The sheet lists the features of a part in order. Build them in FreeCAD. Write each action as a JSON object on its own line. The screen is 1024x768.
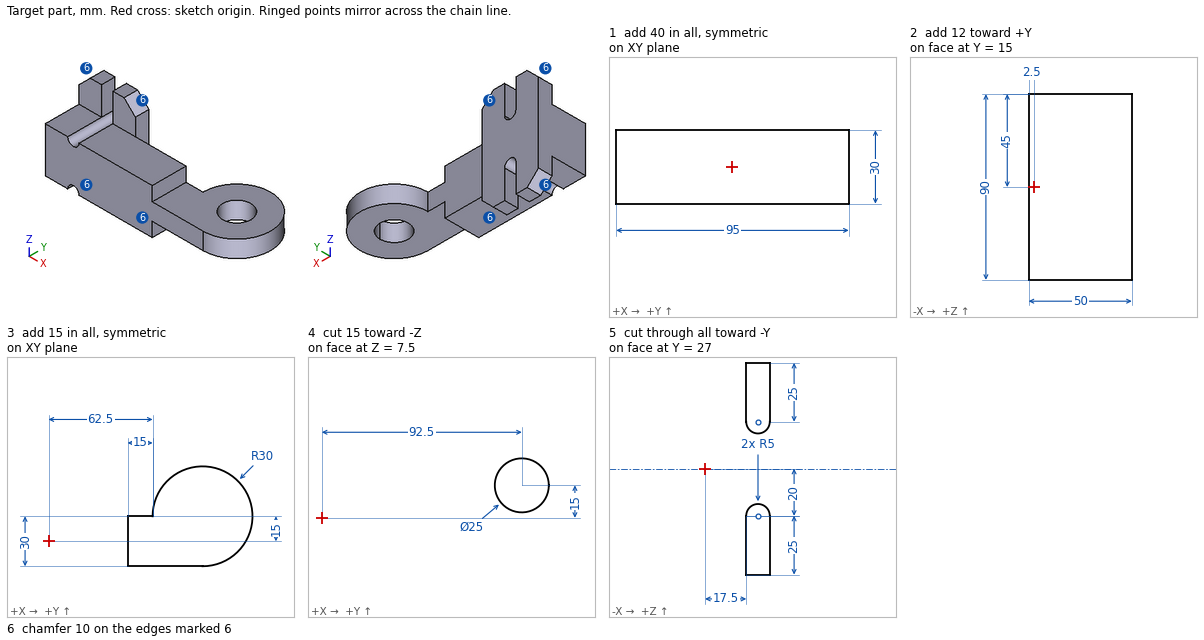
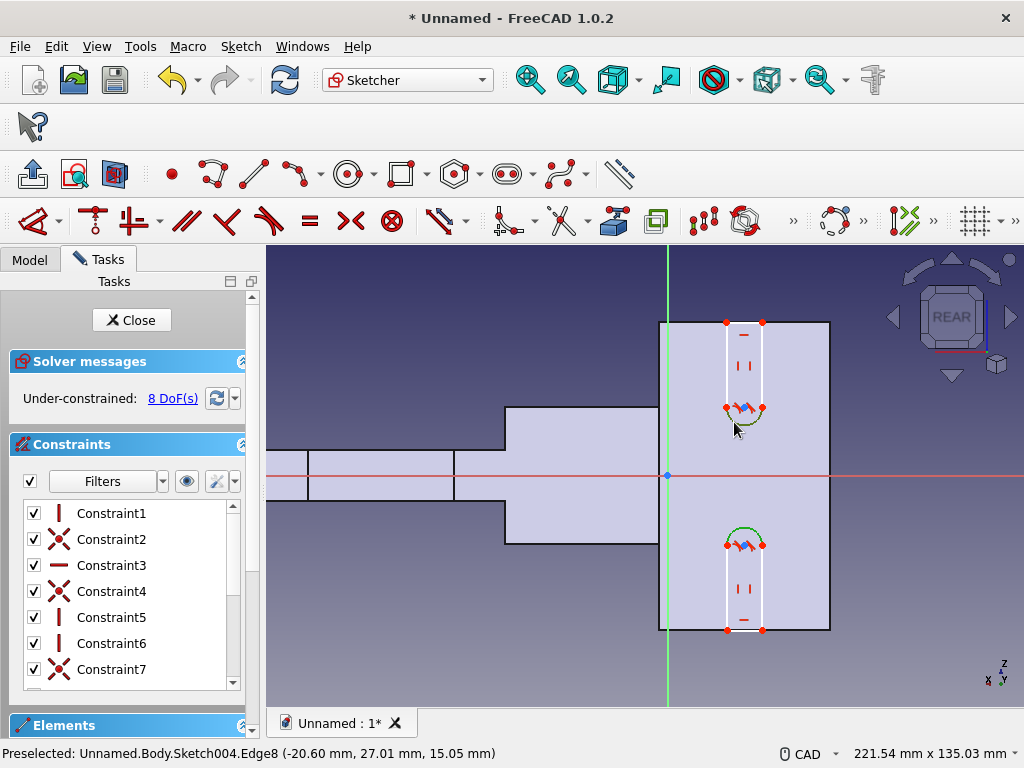
{"action": "left_click", "coordinate": [310, 222]}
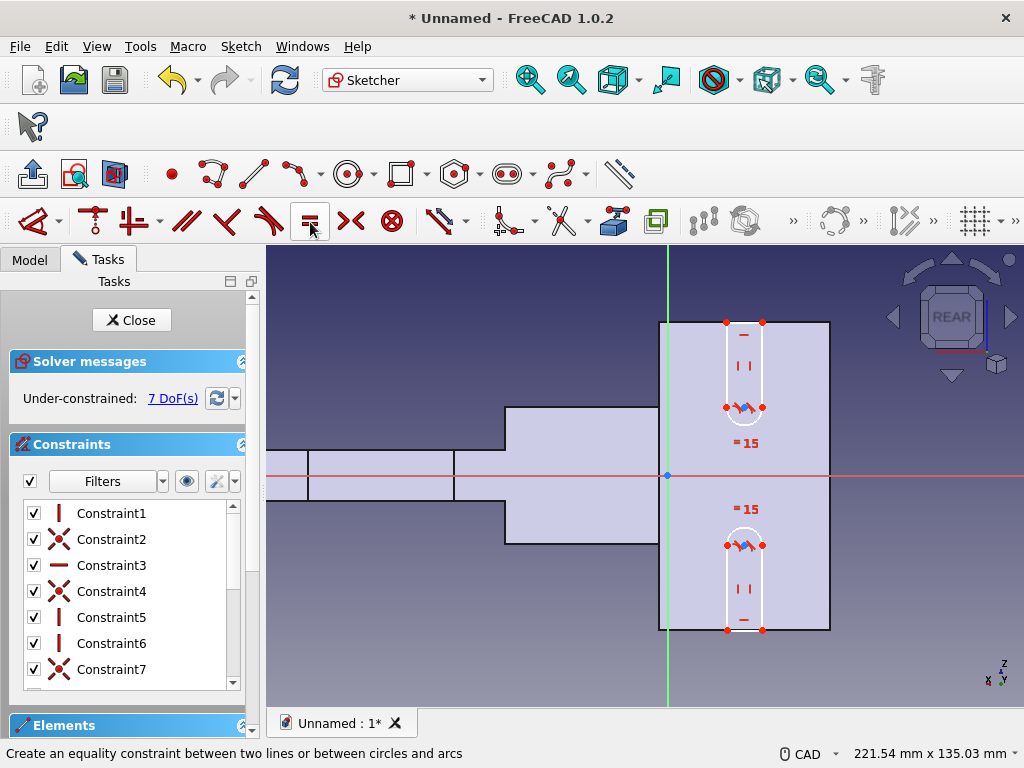
{"action": "left_click", "coordinate": [745, 545]}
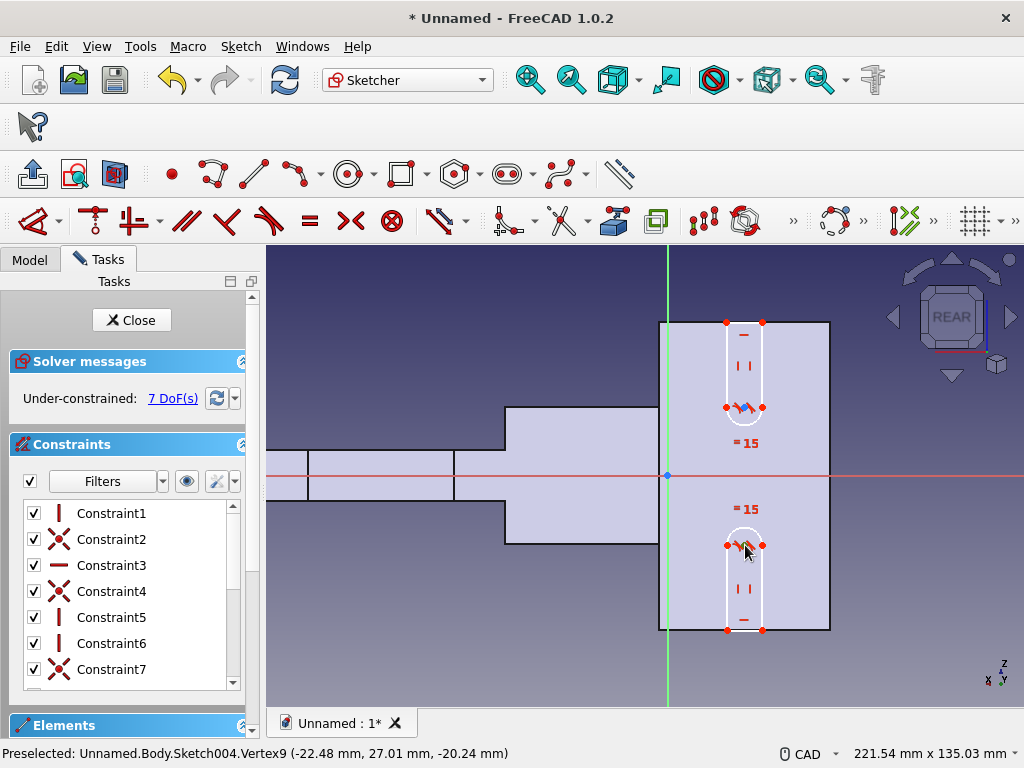
{"action": "left_click", "coordinate": [744, 408]}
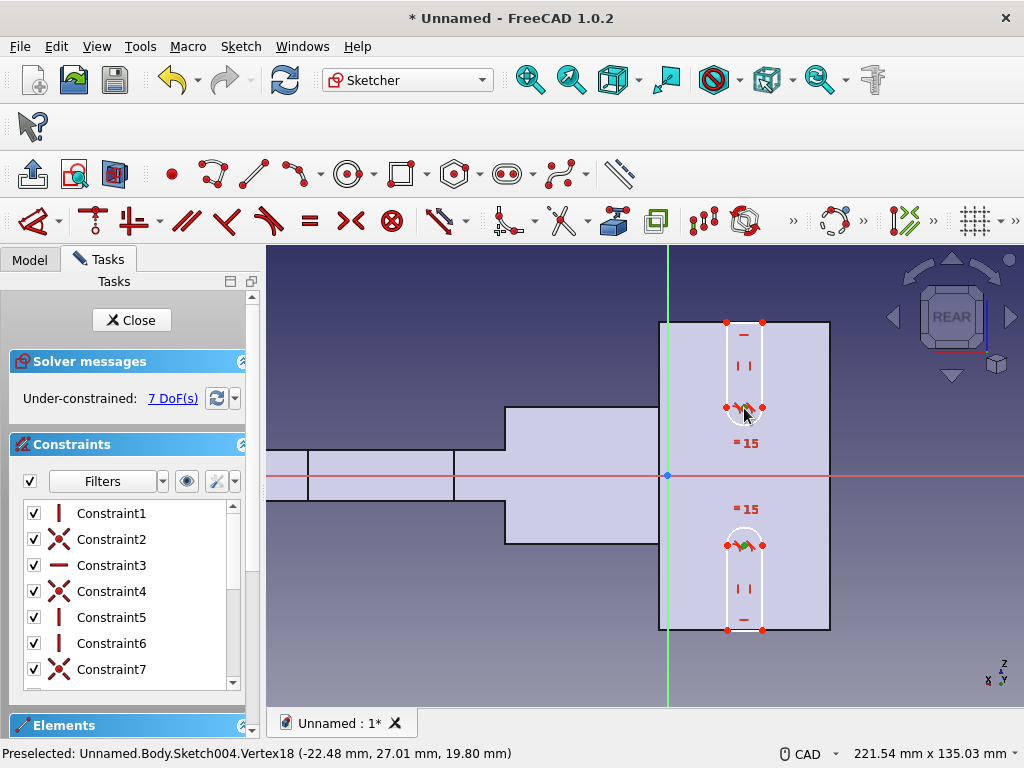
{"action": "left_click", "coordinate": [334, 476]}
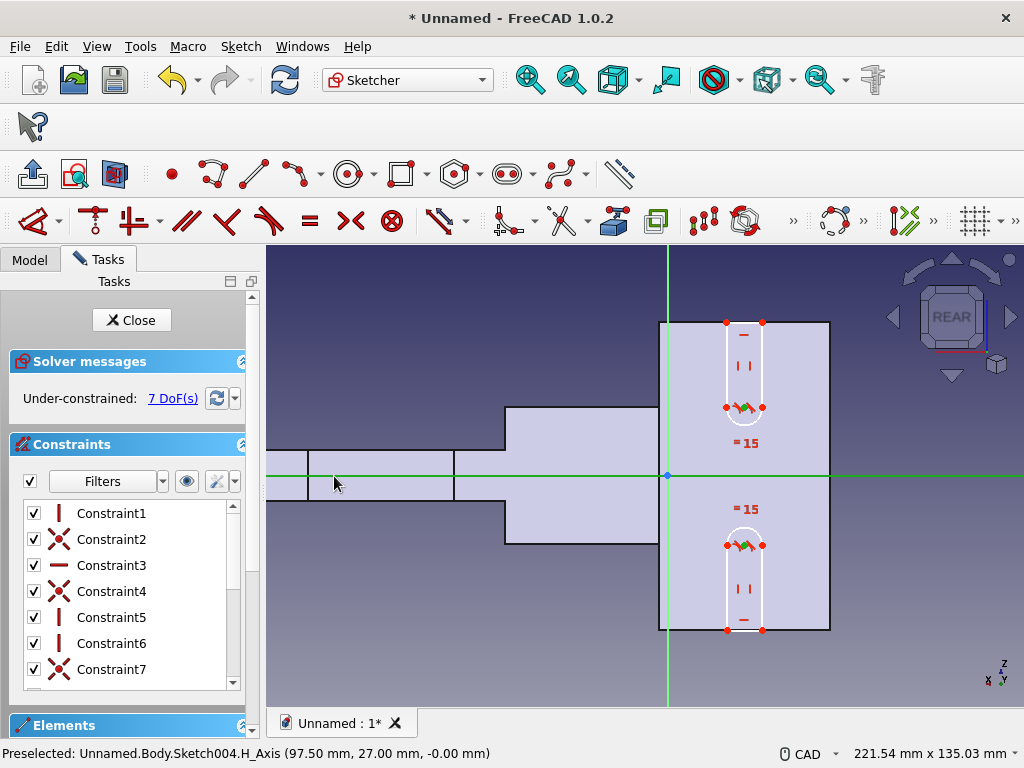
{"action": "key", "text": "s"}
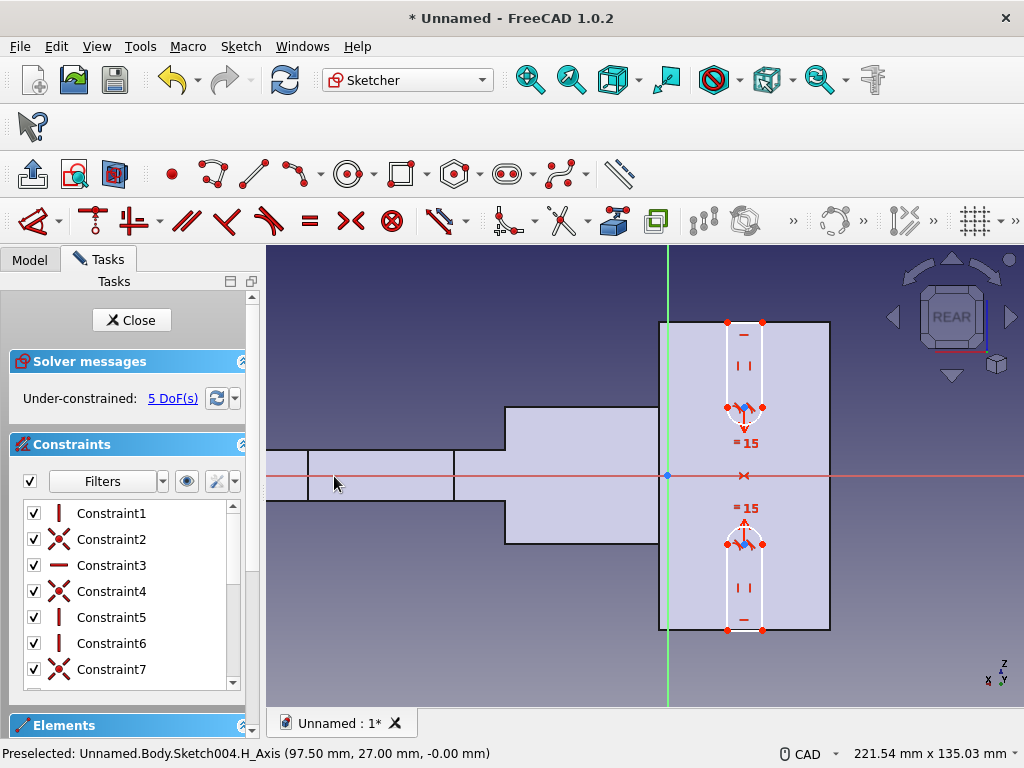
{"action": "left_click", "coordinate": [32, 222]}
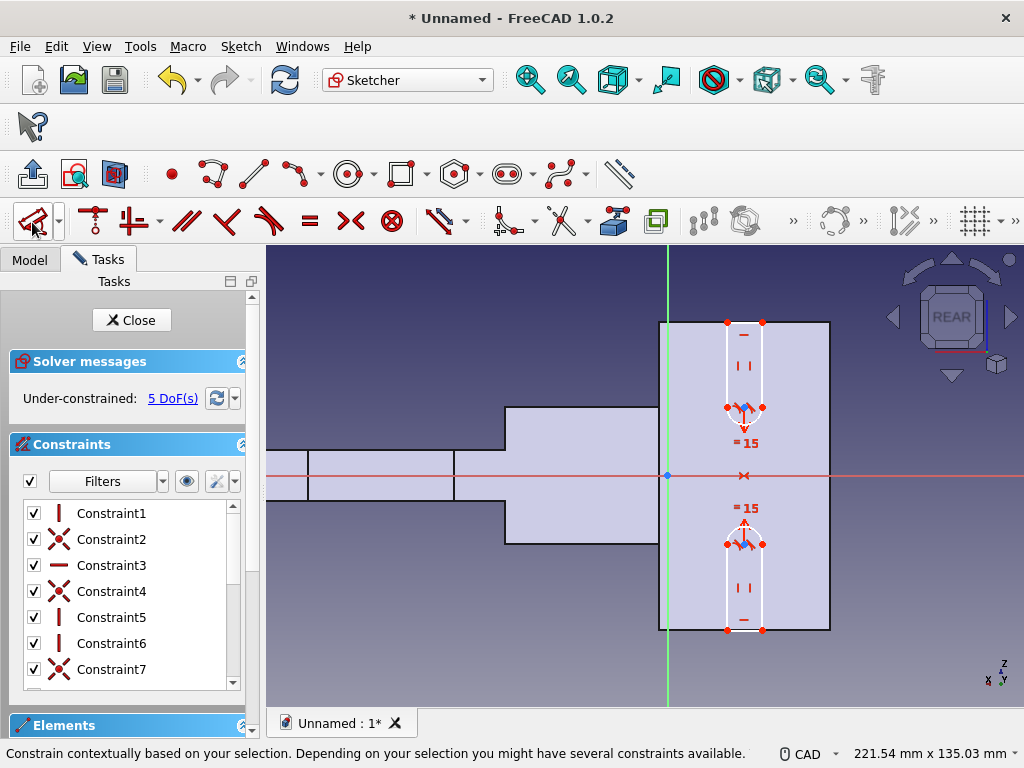
{"action": "scroll", "coordinate": [755, 530], "scroll_direction": "up", "scroll_amount": 5}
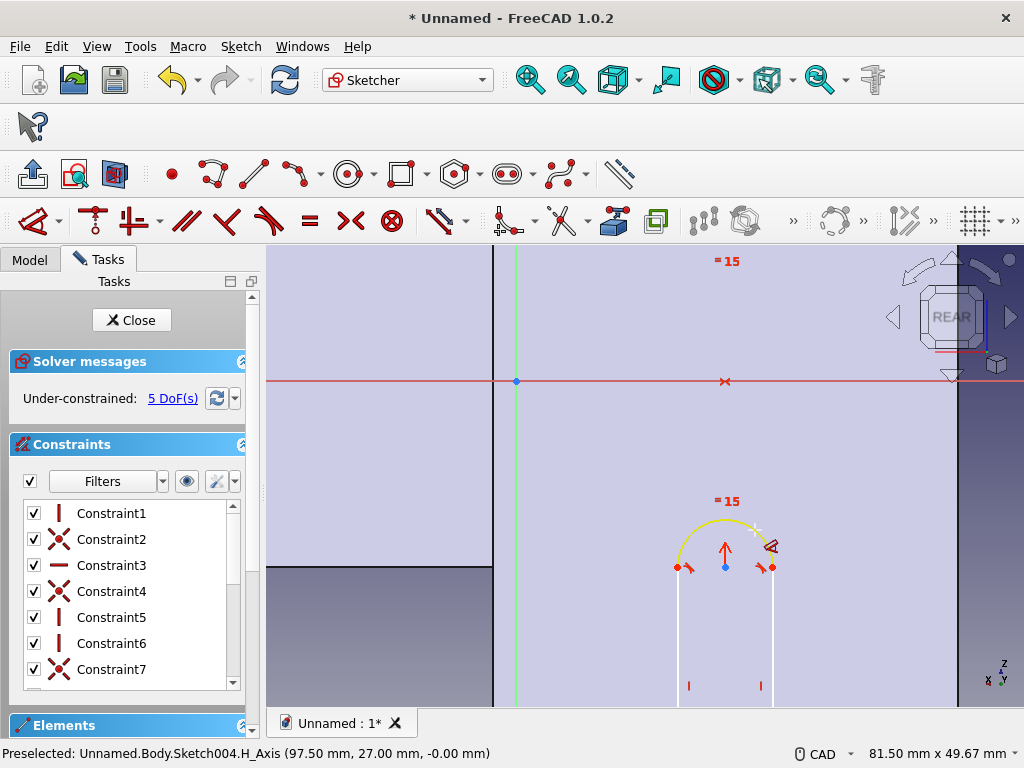
{"action": "left_click", "coordinate": [753, 529]}
{"action": "left_click", "coordinate": [772, 503]}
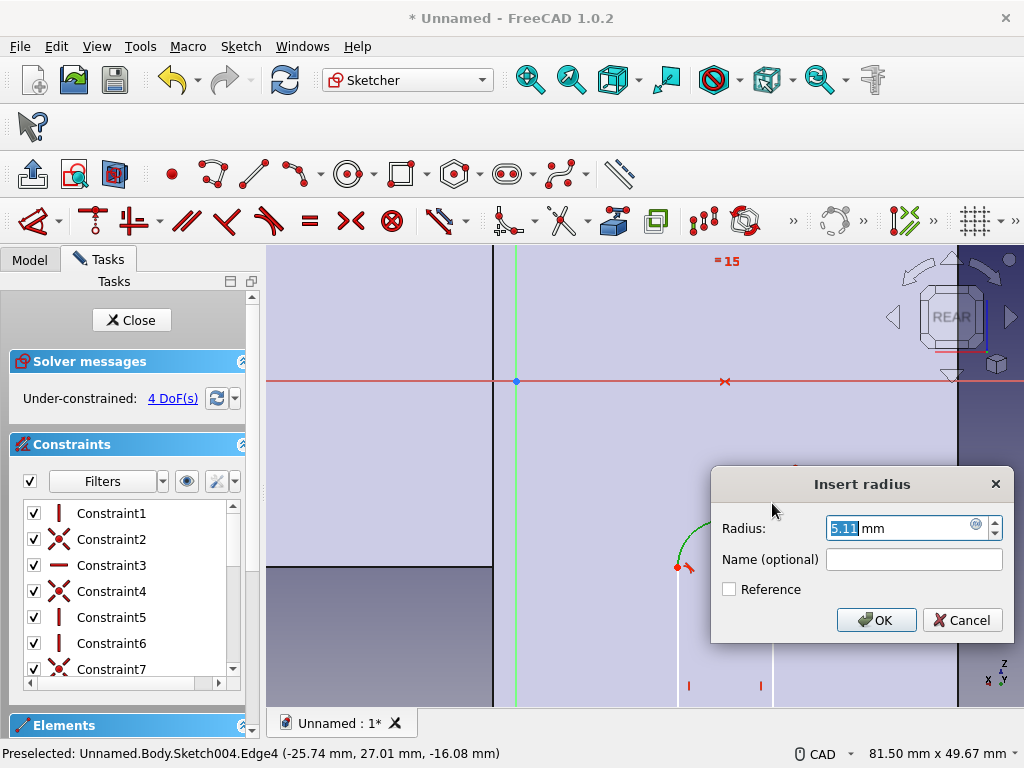
{"action": "type", "text": "5"}
{"action": "key", "text": "Return"}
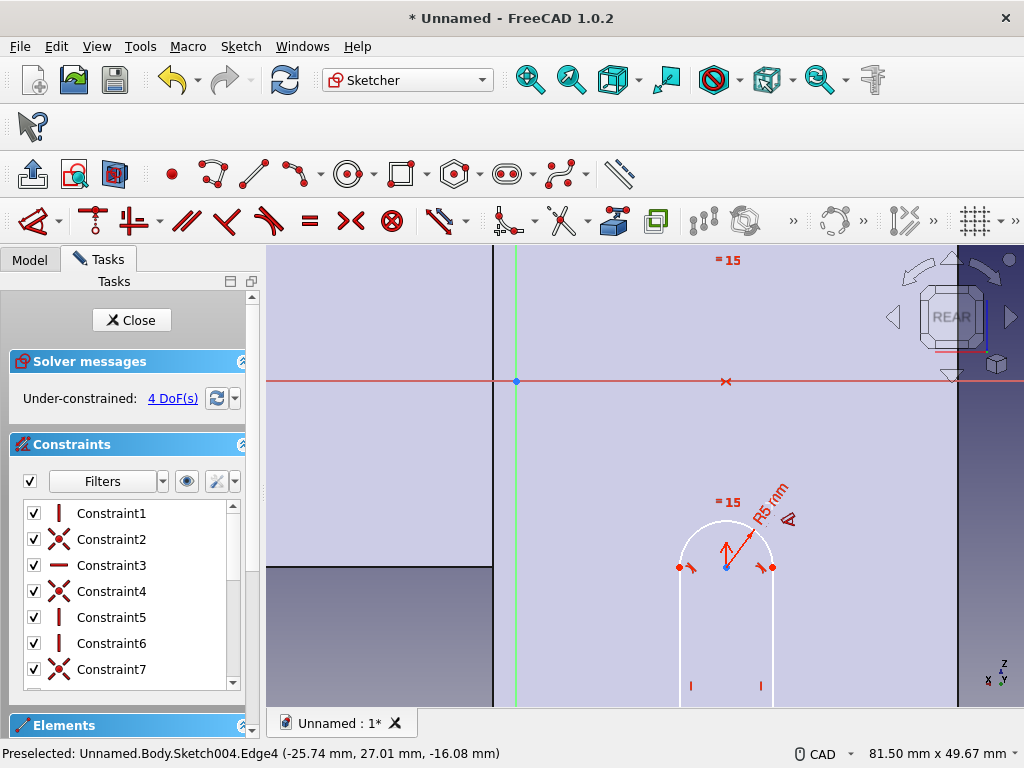
{"action": "left_click", "coordinate": [680, 638]}
{"action": "left_click", "coordinate": [714, 623]}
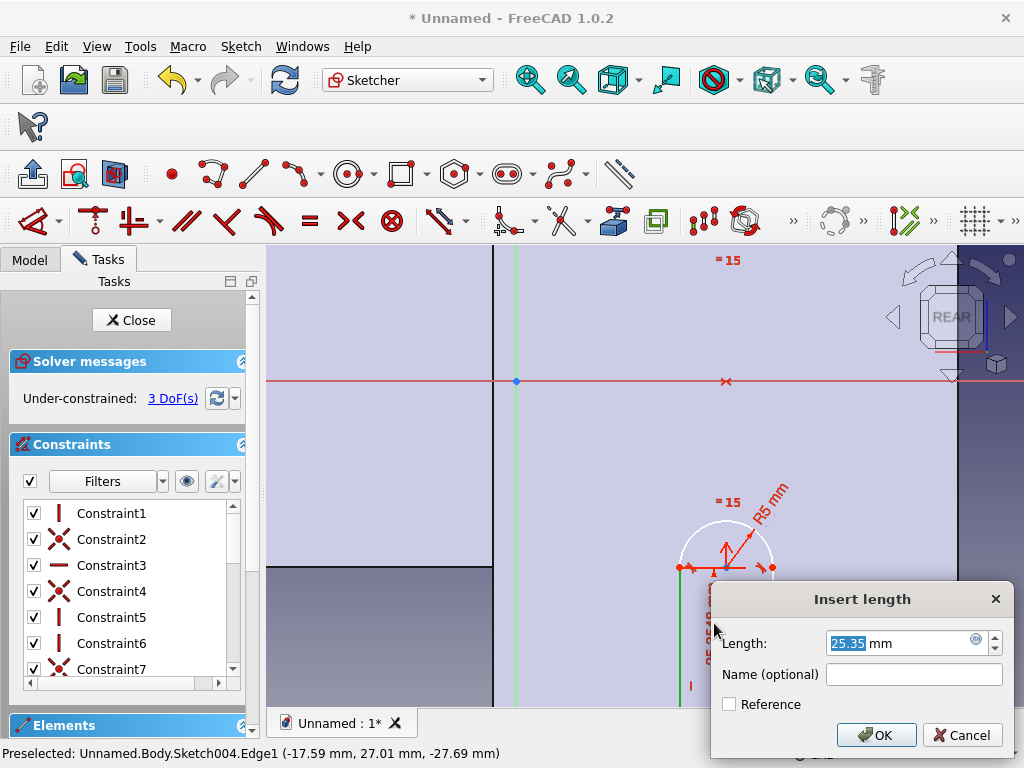
{"action": "type", "text": "25"}
{"action": "key", "text": "Return"}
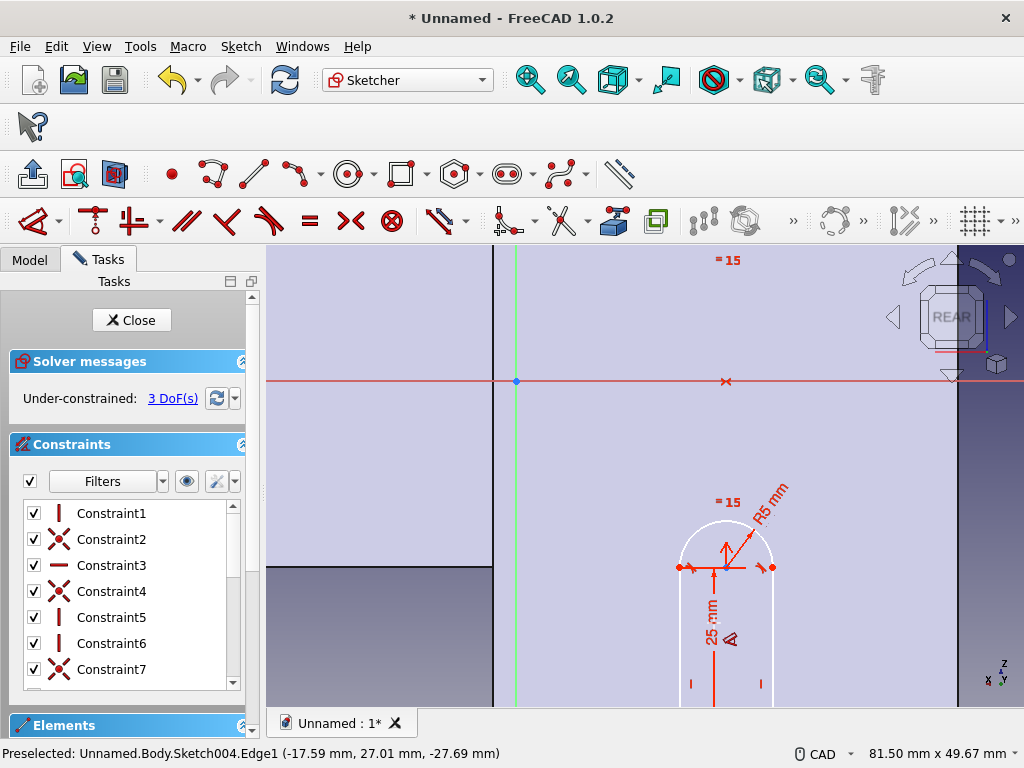
{"action": "scroll", "coordinate": [537, 531], "scroll_direction": "down", "scroll_amount": 5}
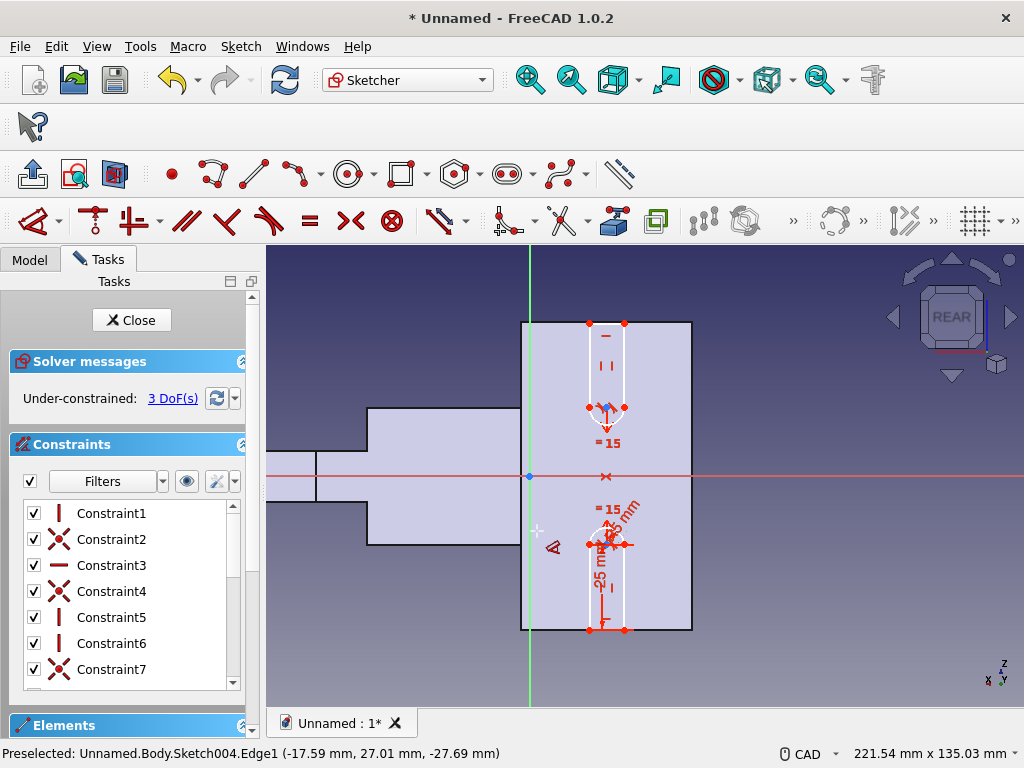
{"action": "left_click", "coordinate": [624, 383]}
{"action": "left_click", "coordinate": [658, 366]}